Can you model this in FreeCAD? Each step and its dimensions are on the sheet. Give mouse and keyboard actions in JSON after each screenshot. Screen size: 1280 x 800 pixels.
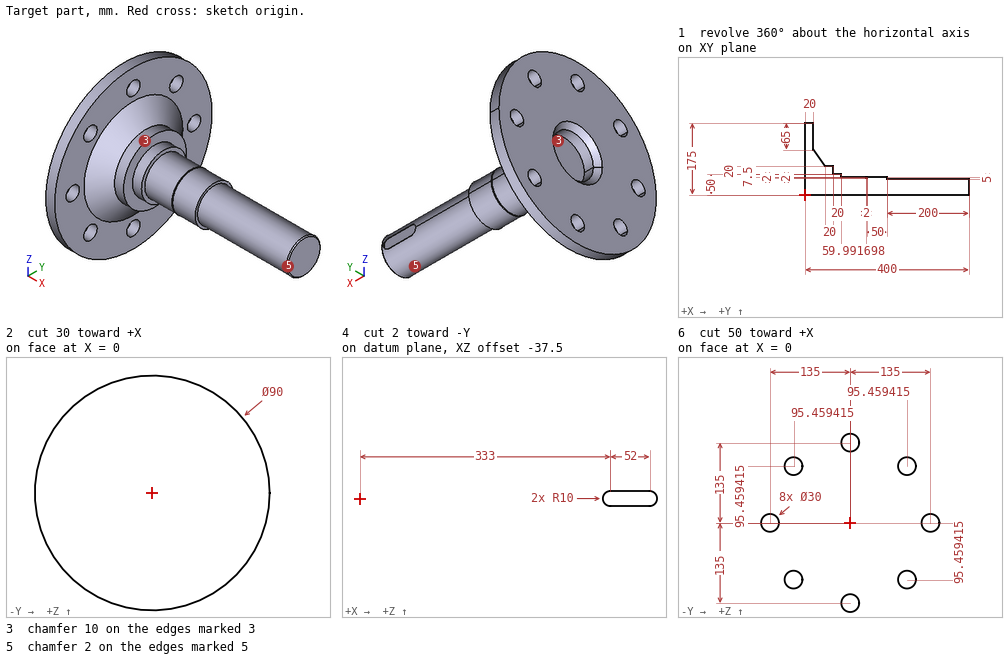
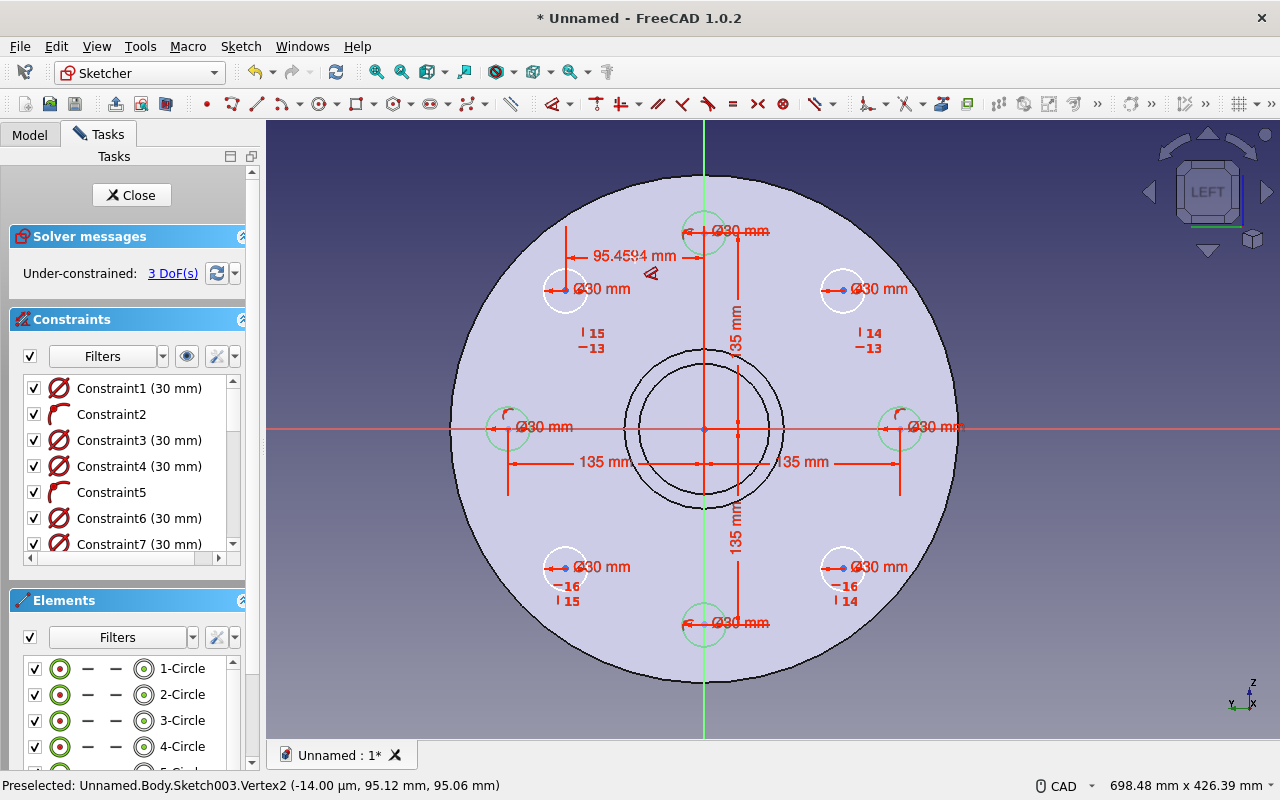
{"action": "left_click", "coordinate": [566, 291]}
{"action": "left_click", "coordinate": [532, 360]}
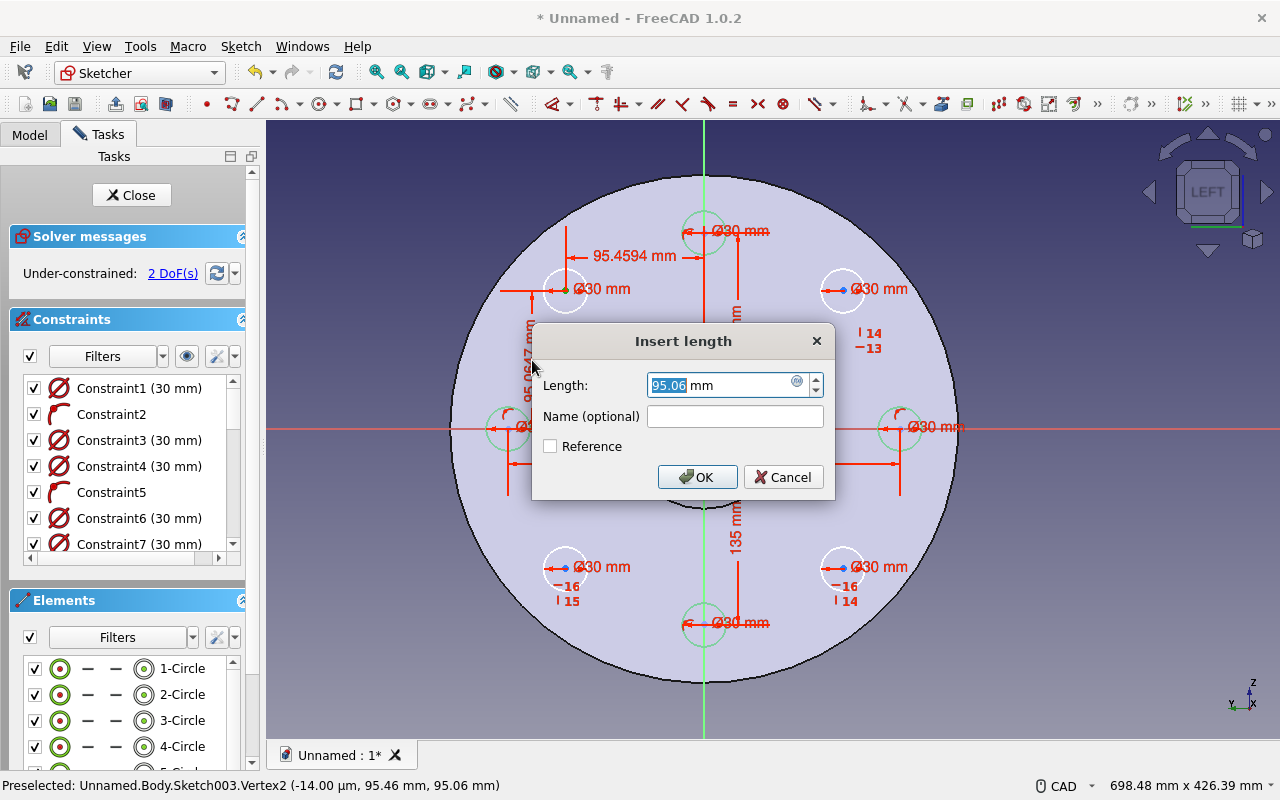
{"action": "type", "text": "95.459415"}
{"action": "key", "text": "Return"}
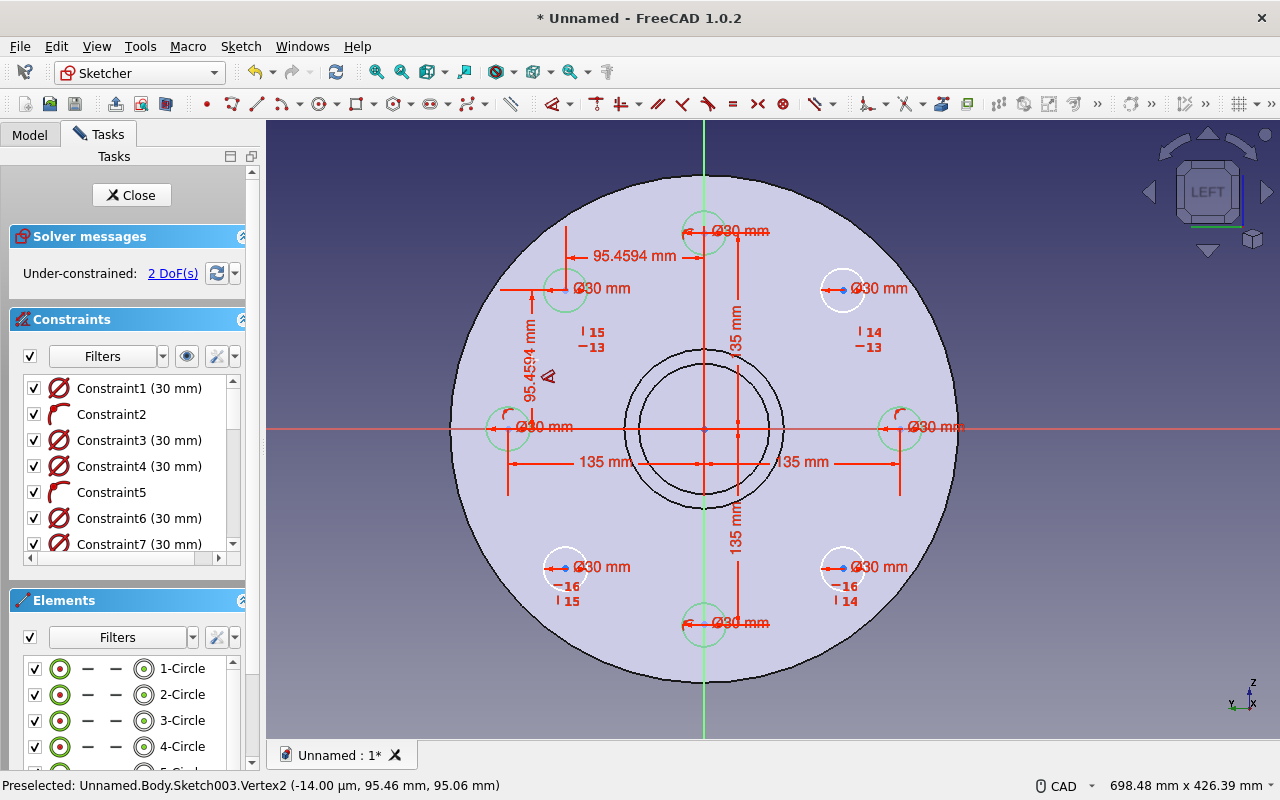
{"action": "left_click", "coordinate": [843, 290]}
{"action": "left_click", "coordinate": [774, 256]}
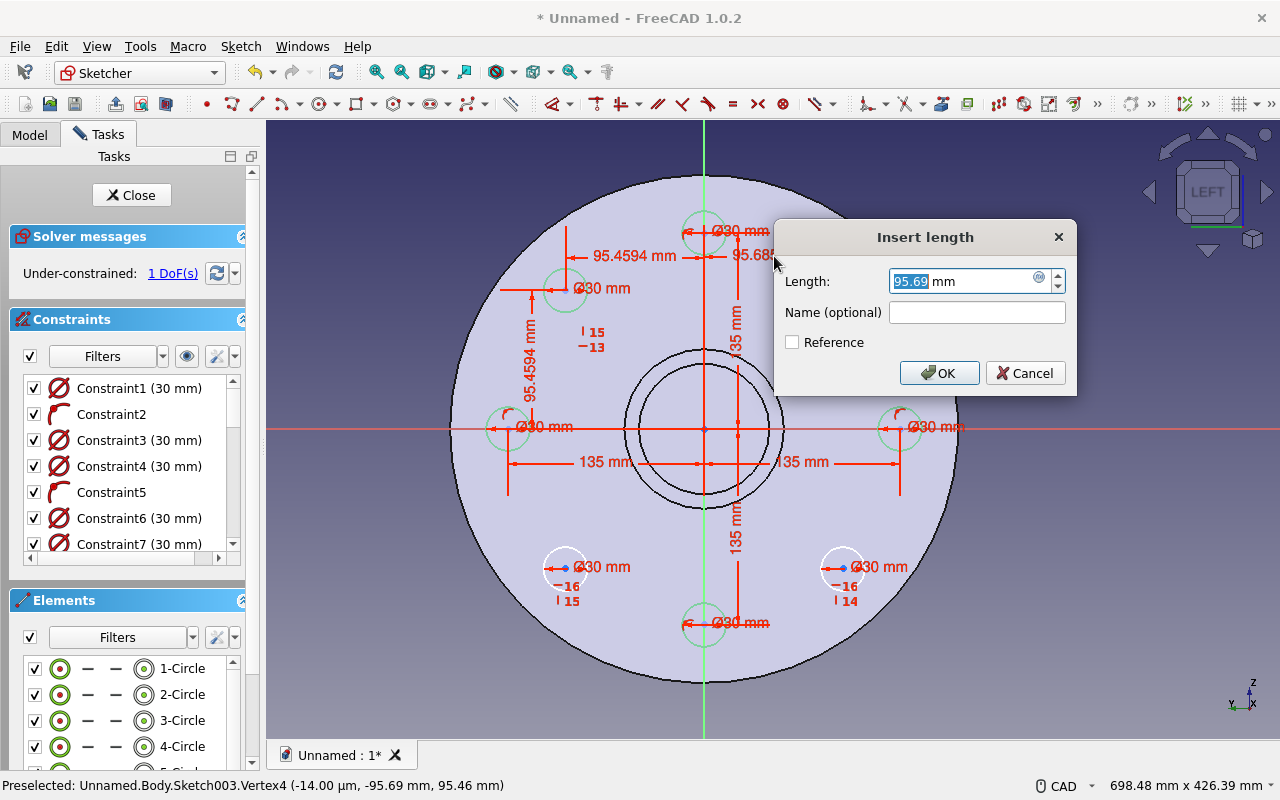
{"action": "type", "text": "95.459415"}
{"action": "key", "text": "Return"}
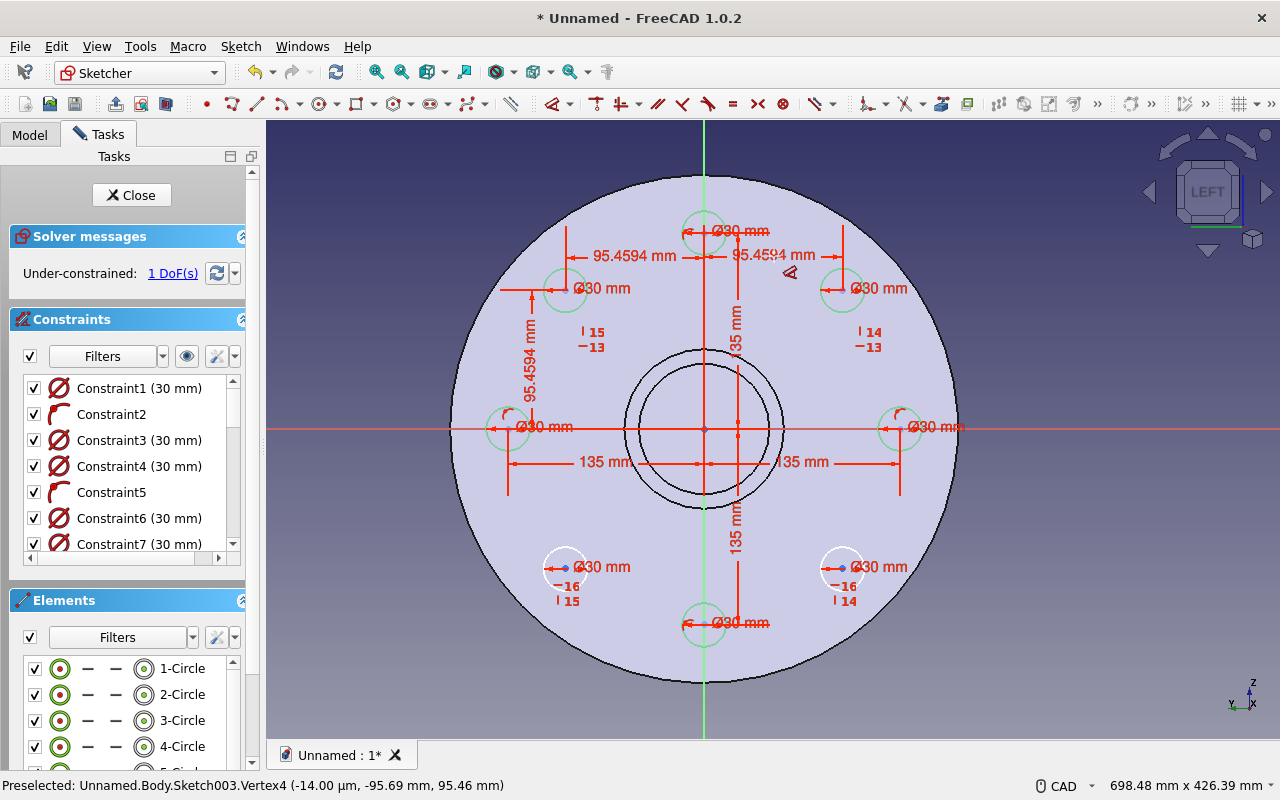
{"action": "left_click", "coordinate": [843, 569]}
{"action": "left_click", "coordinate": [877, 499]}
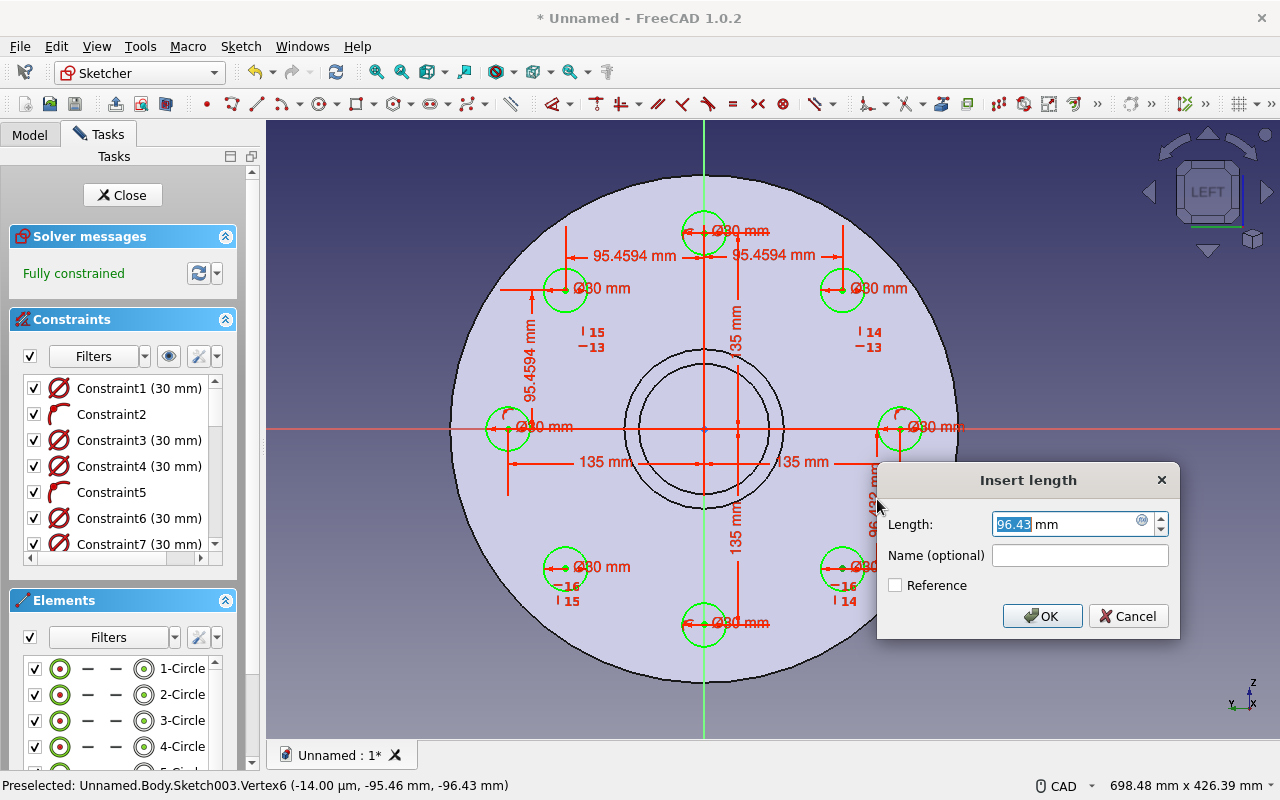
{"action": "type", "text": "95.459415"}
{"action": "key", "text": "Return"}
{"action": "key", "text": "Escape"}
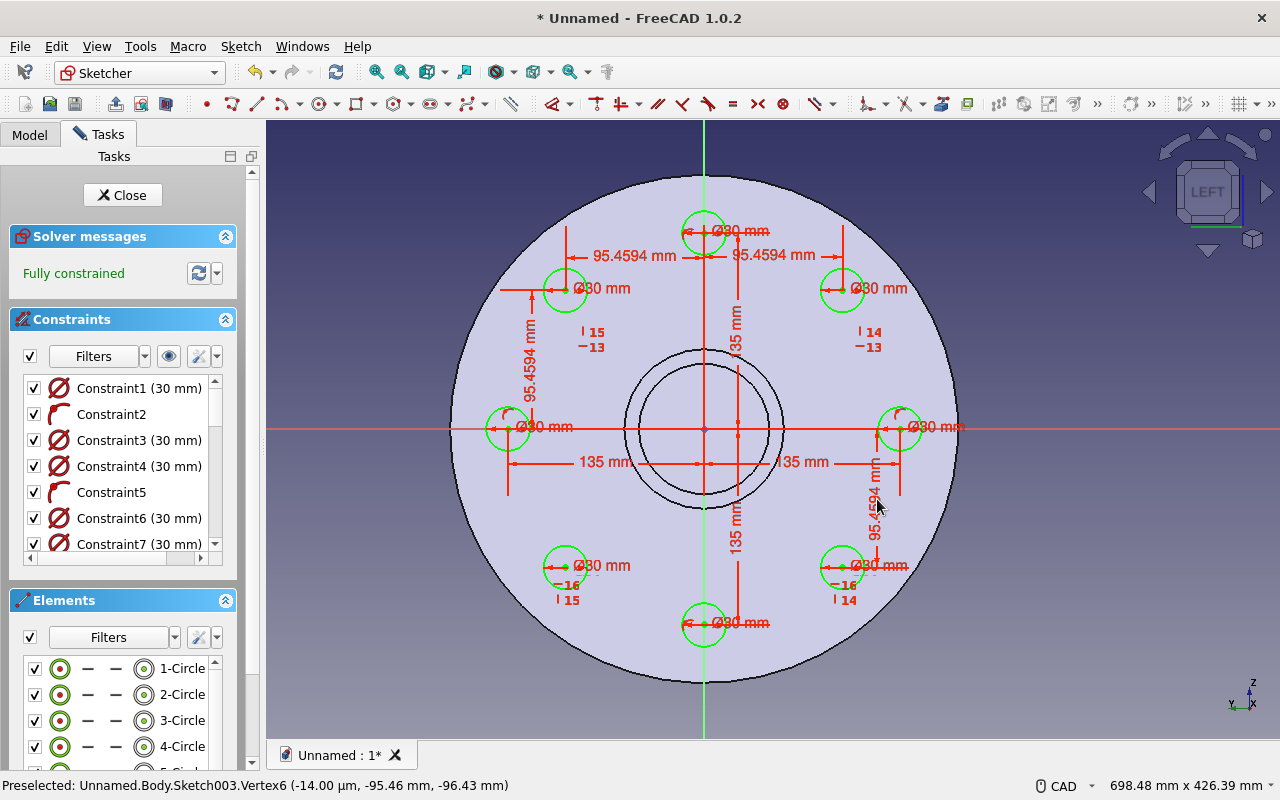
{"action": "left_click", "coordinate": [123, 195]}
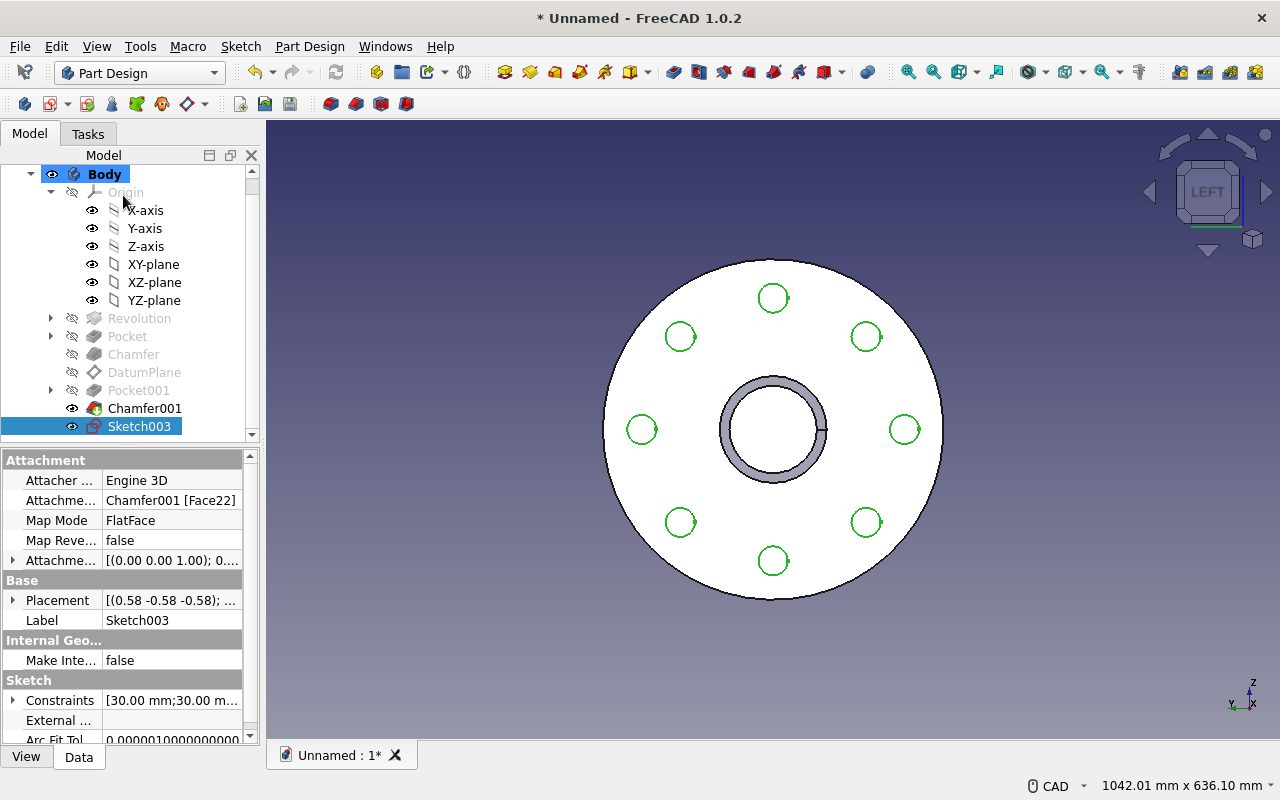
{"action": "left_click", "coordinate": [674, 72]}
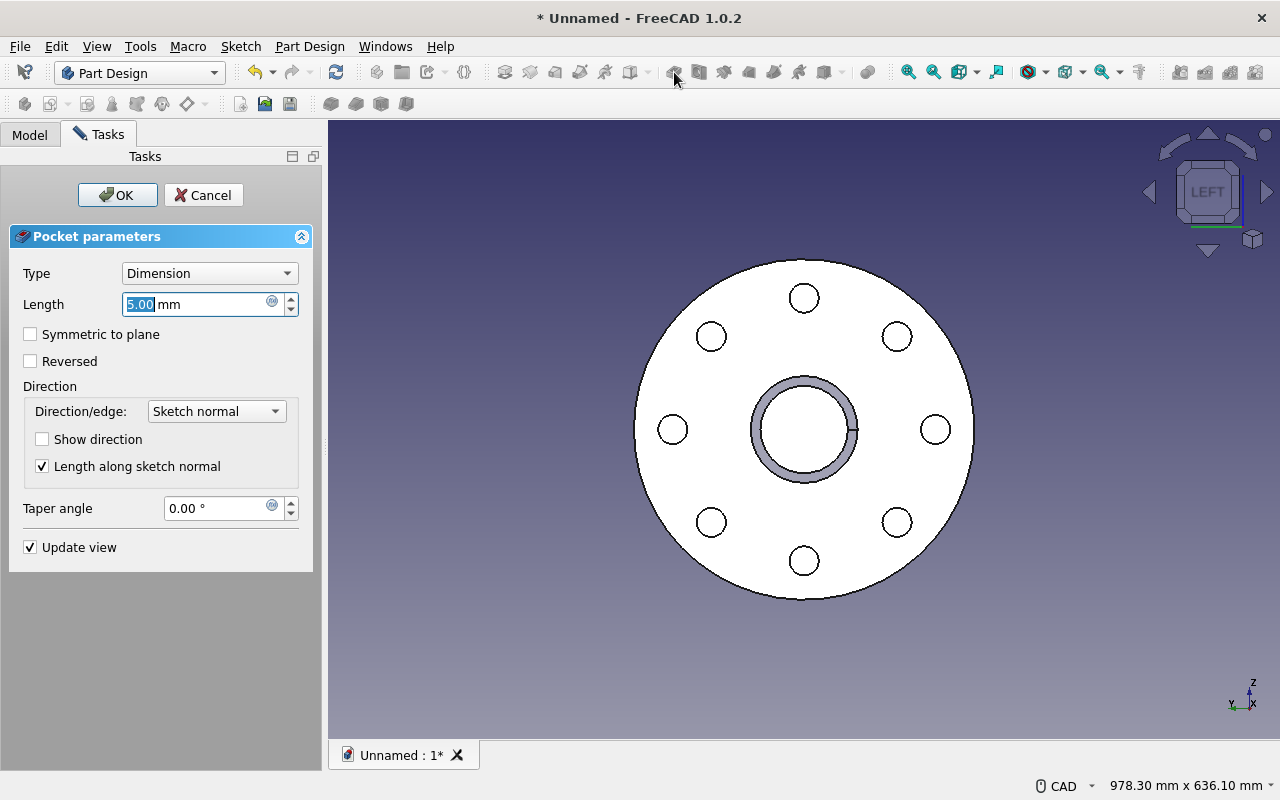
{"action": "type", "text": "50"}
{"action": "key", "text": "Tab"}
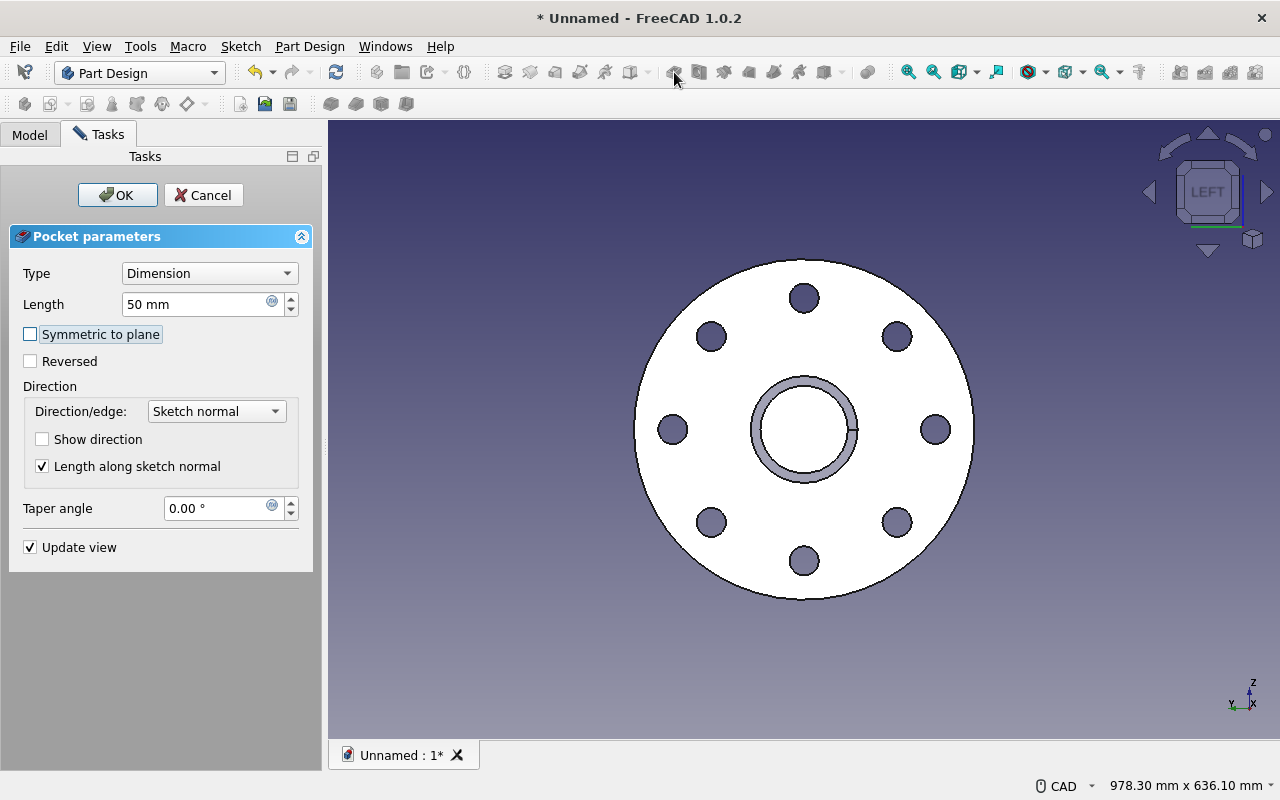
{"action": "left_click", "coordinate": [118, 195]}